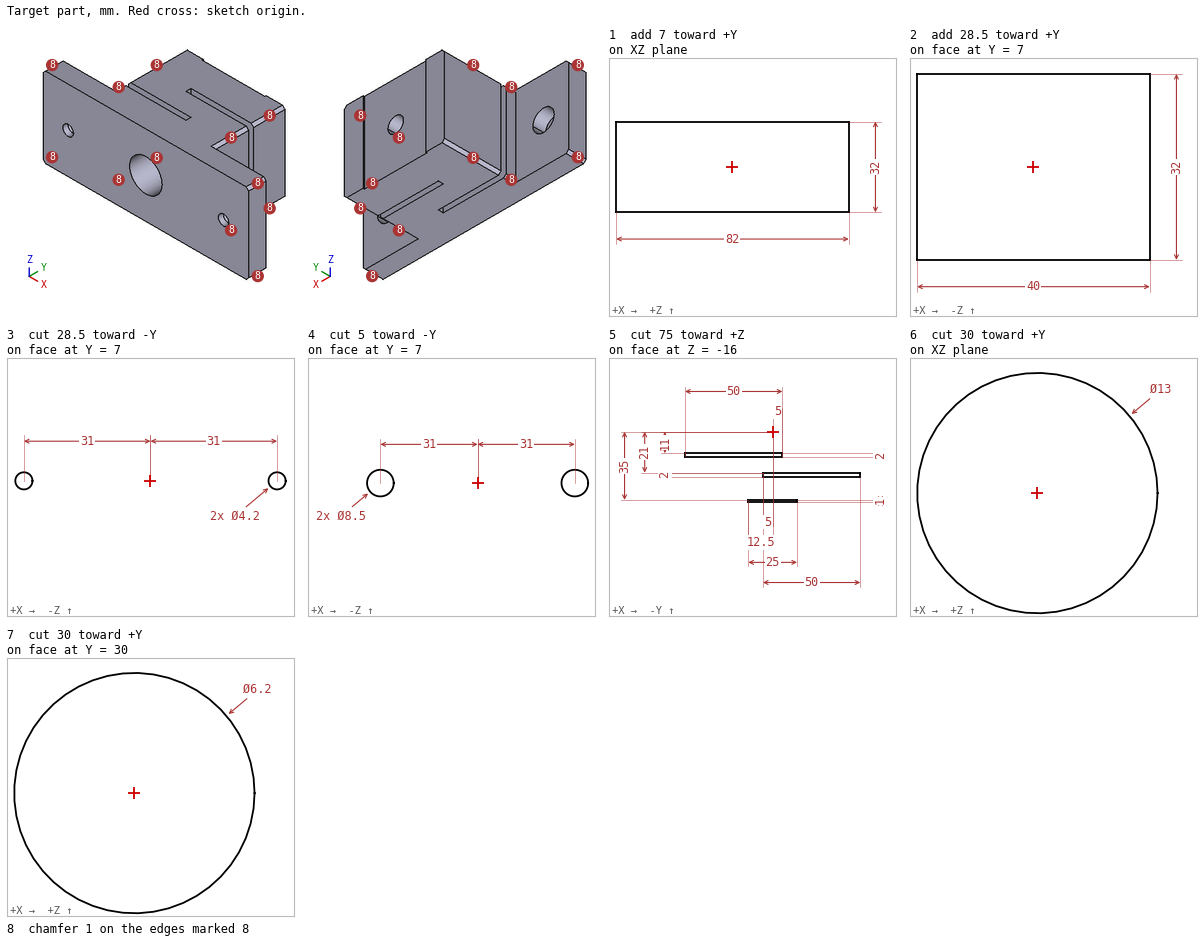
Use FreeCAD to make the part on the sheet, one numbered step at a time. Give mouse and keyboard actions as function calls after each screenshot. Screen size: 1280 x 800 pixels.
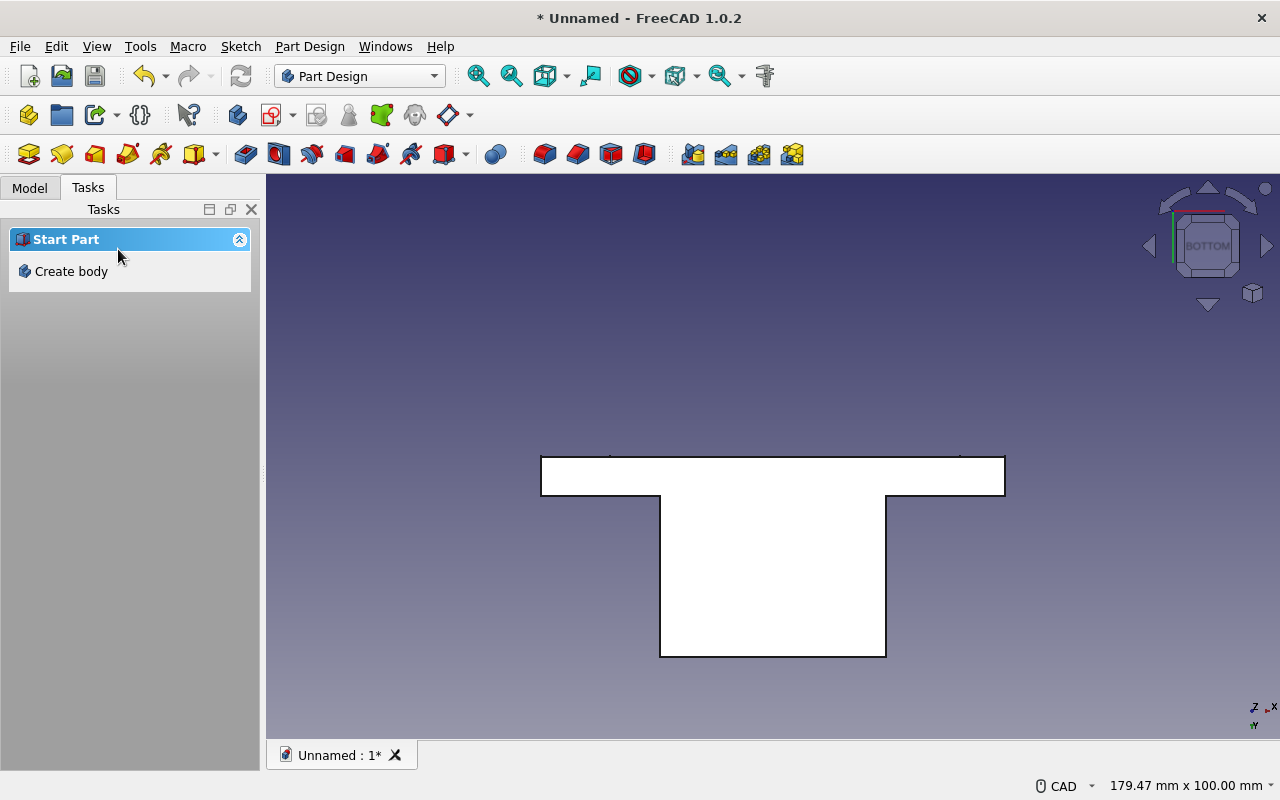
click(773, 556)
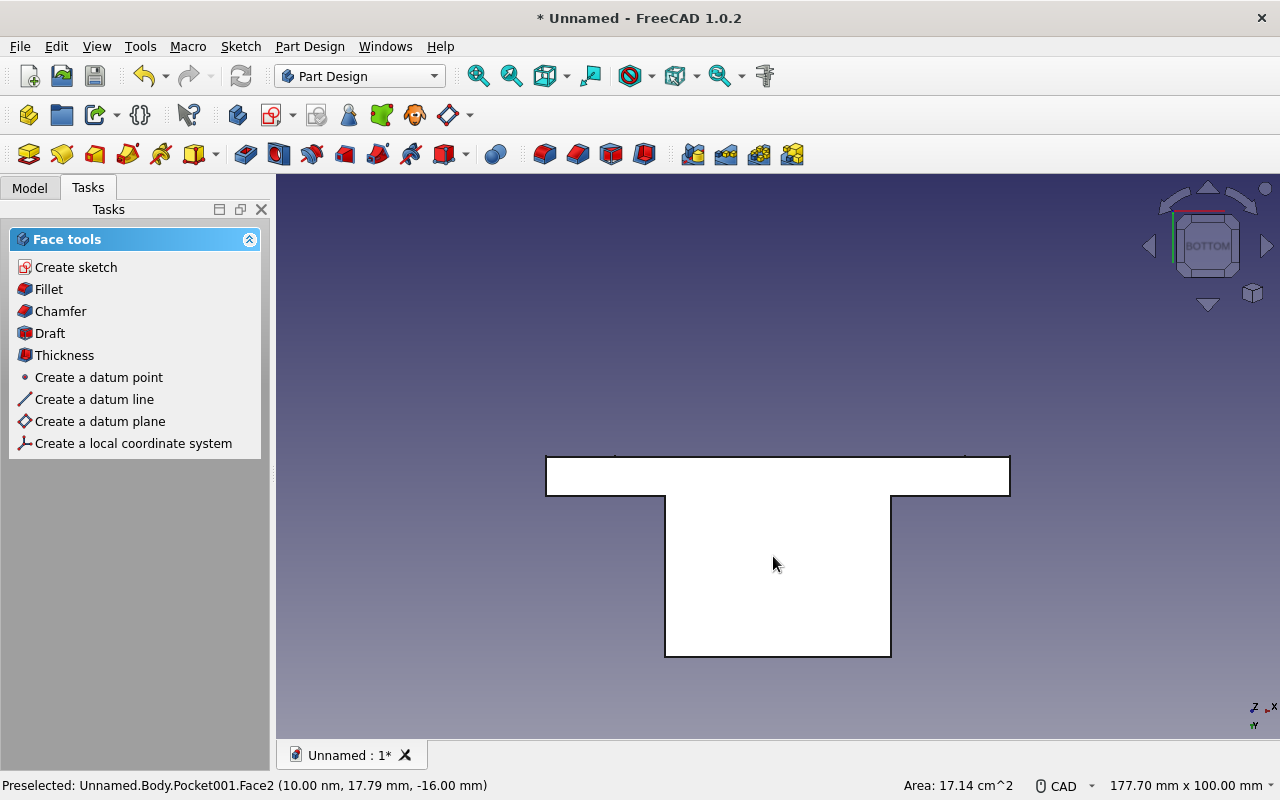
click(270, 116)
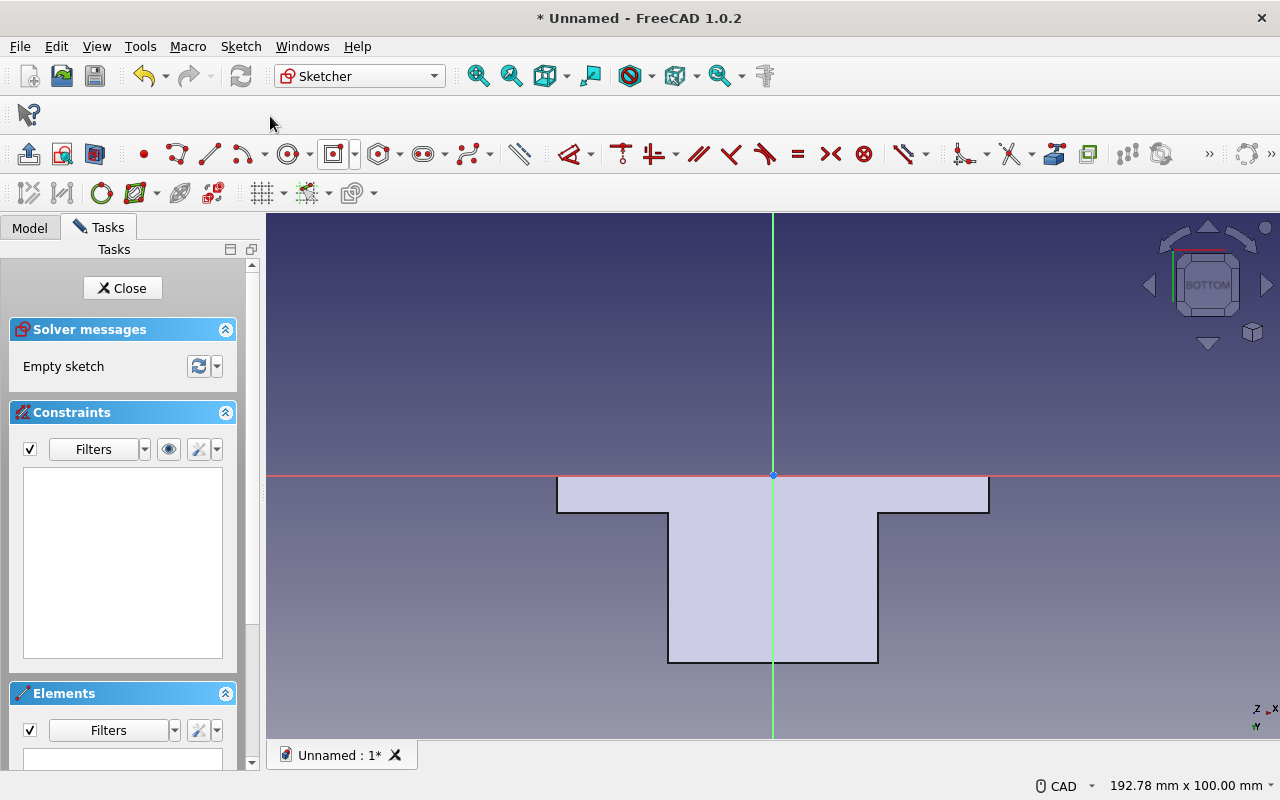
key(g)
key(r)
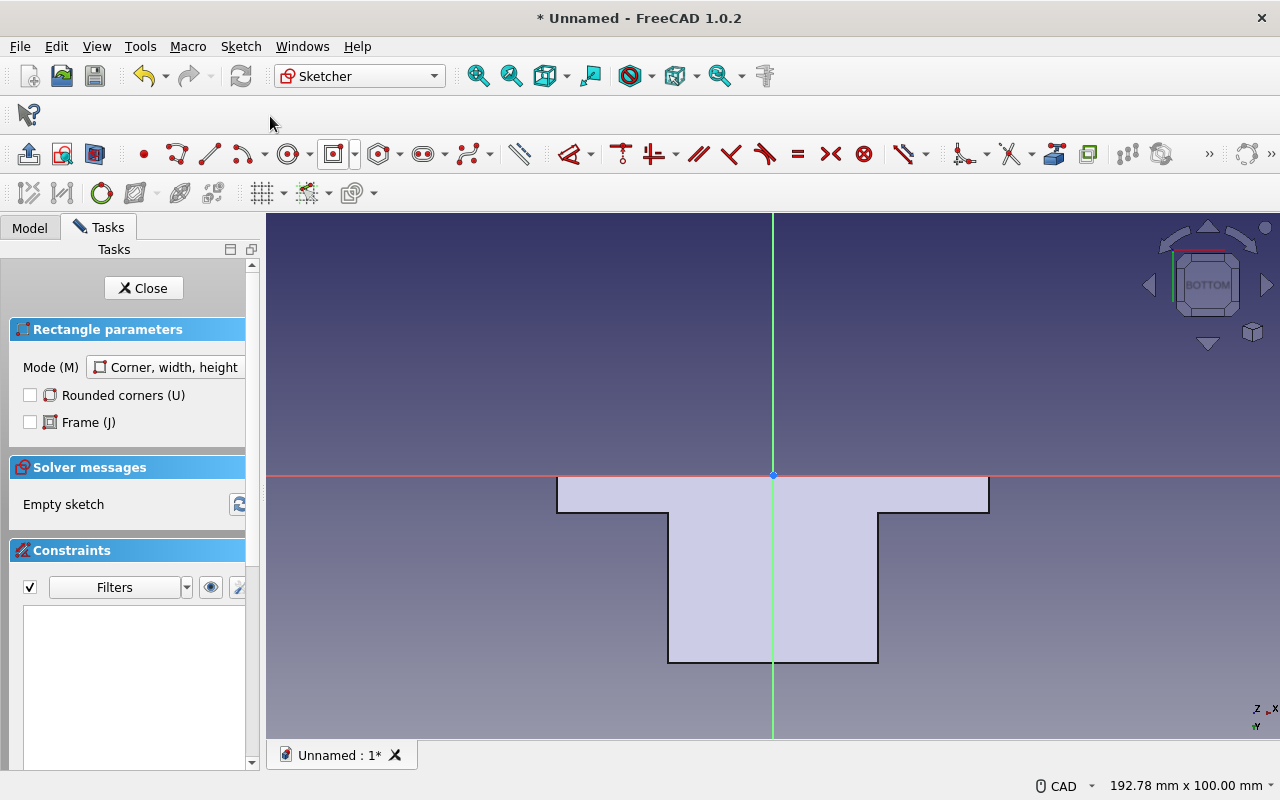
scroll(536, 534, up, 3)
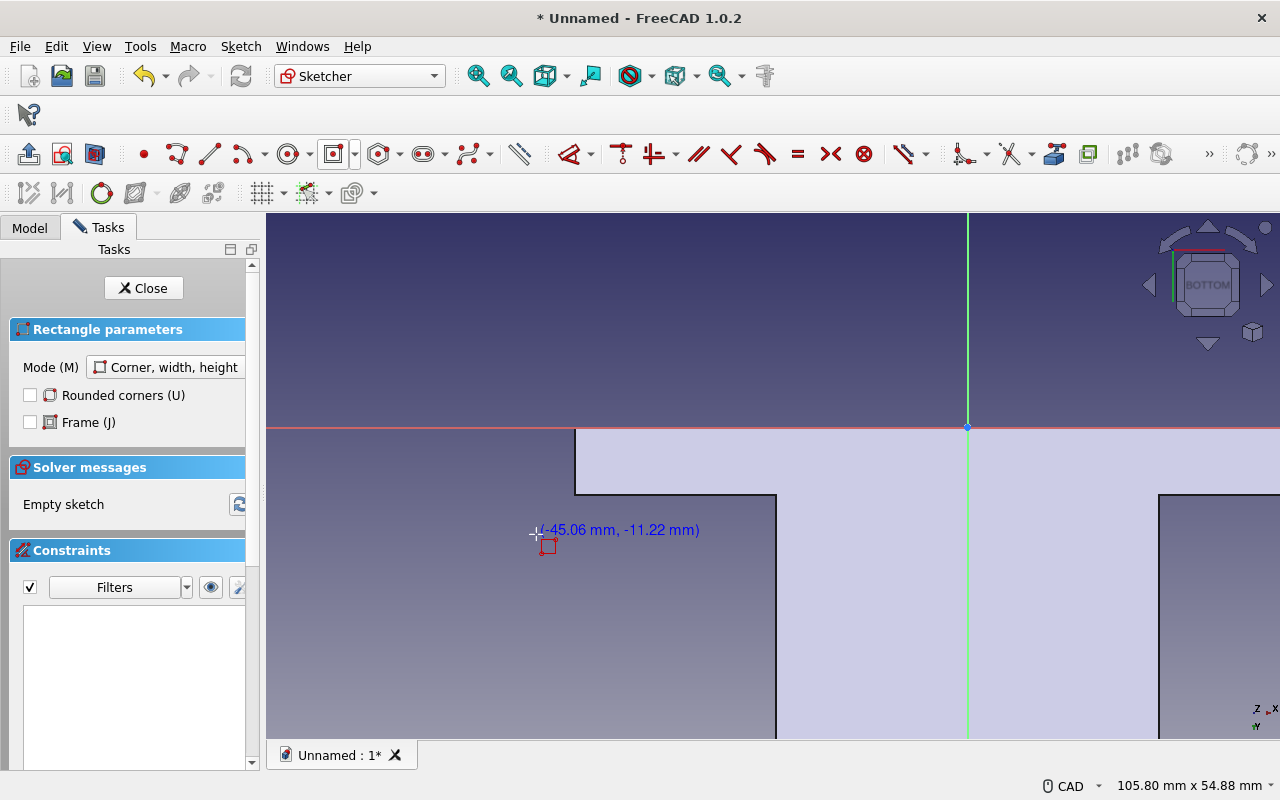
click(536, 533)
move(1016, 552)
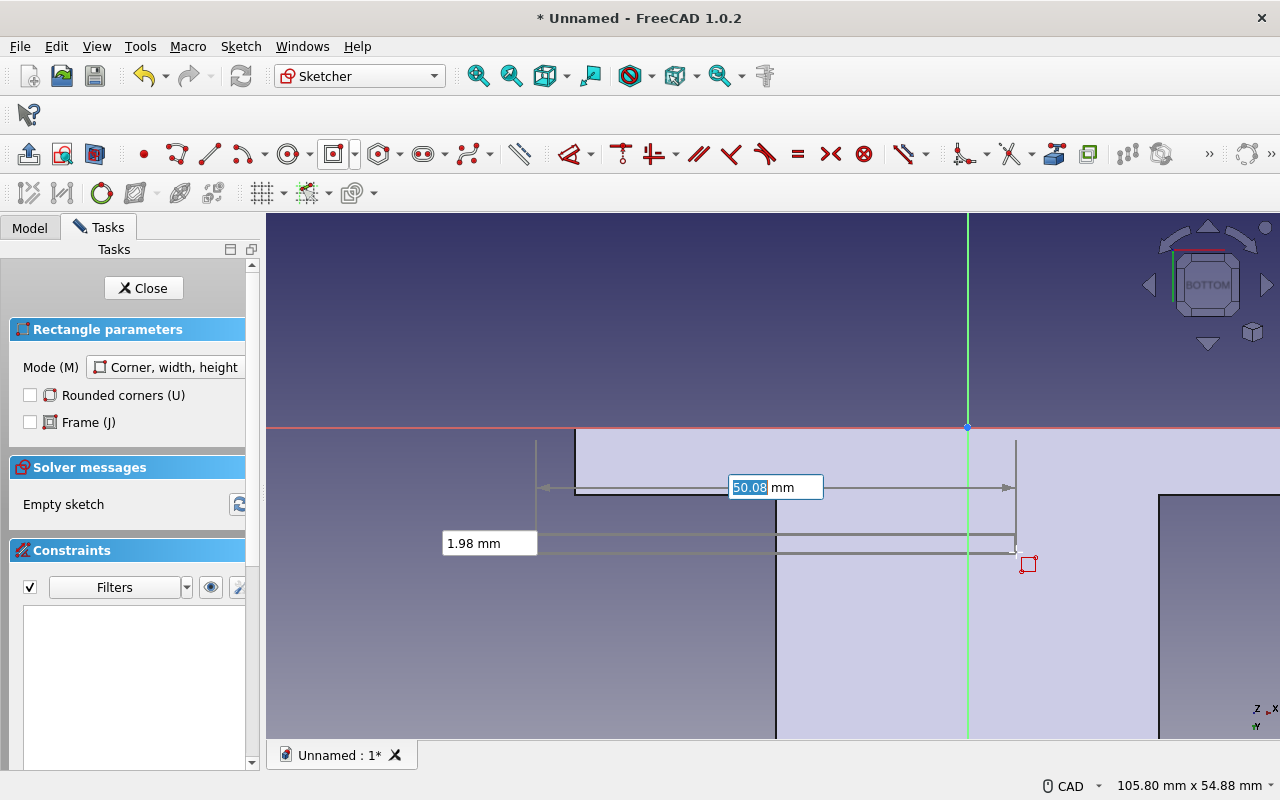
text(50)
key(Tab)
text(2)
key(Return)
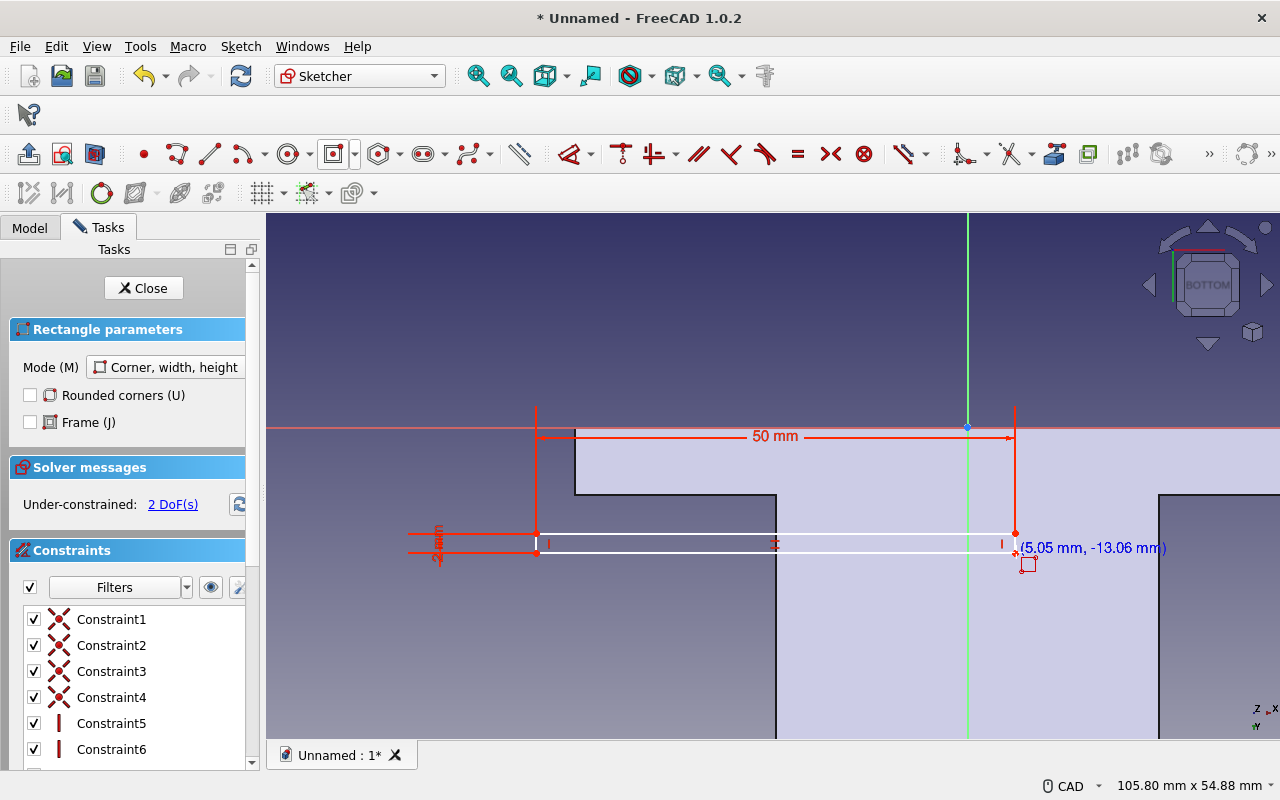
click(920, 629)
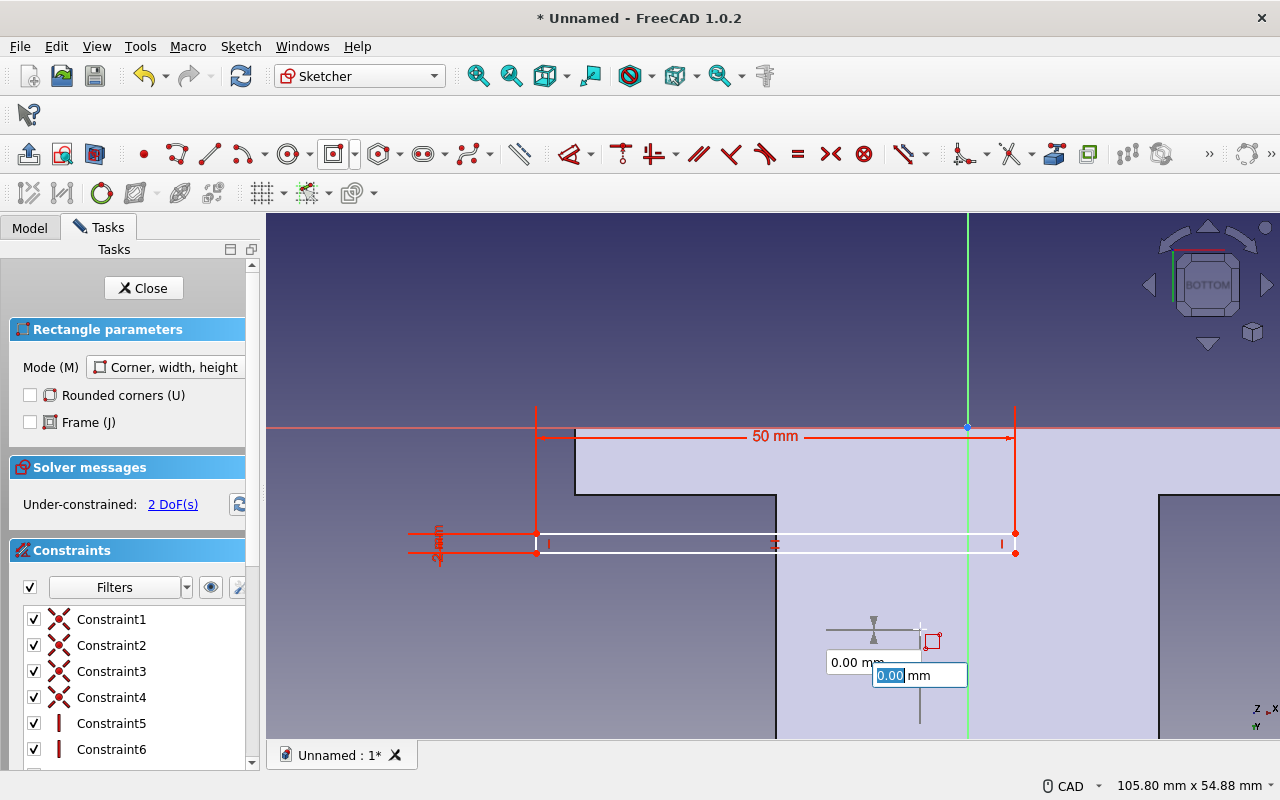
scroll(294, 241, down, 2)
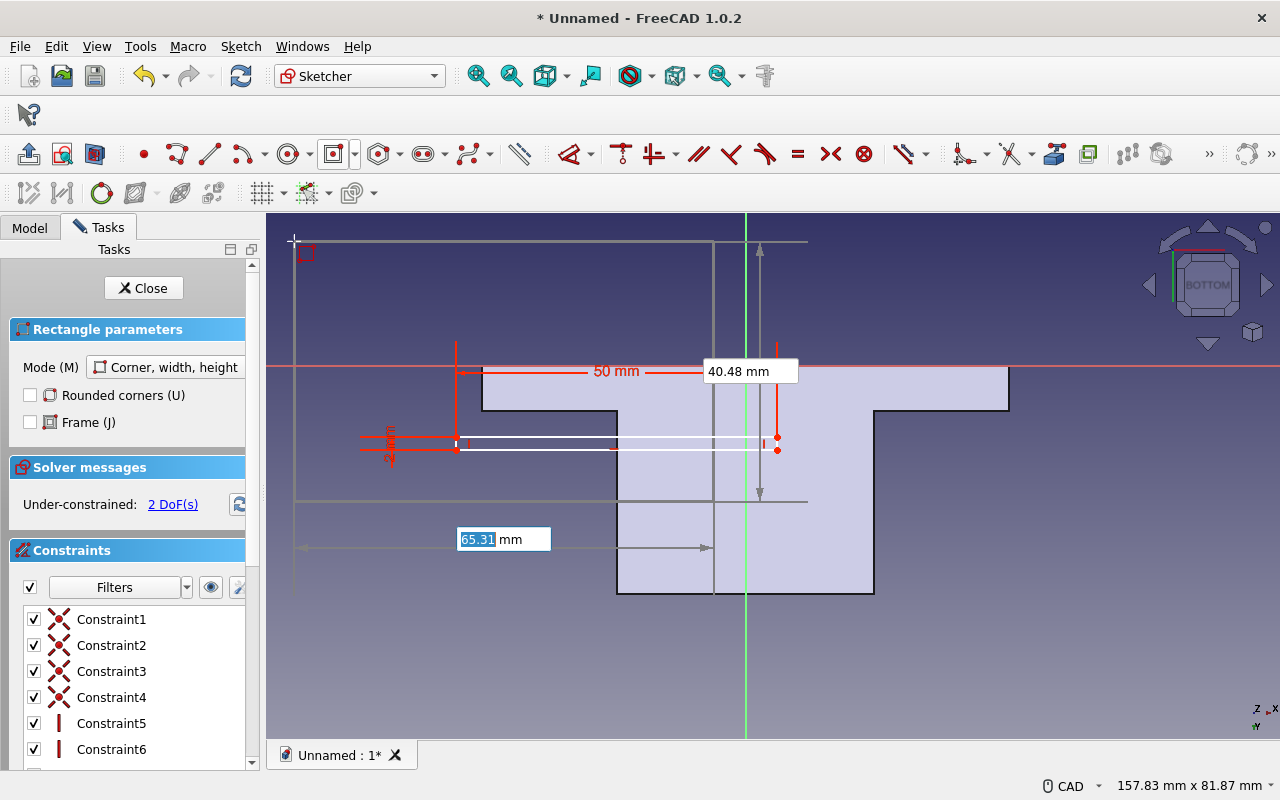
click(1035, 514)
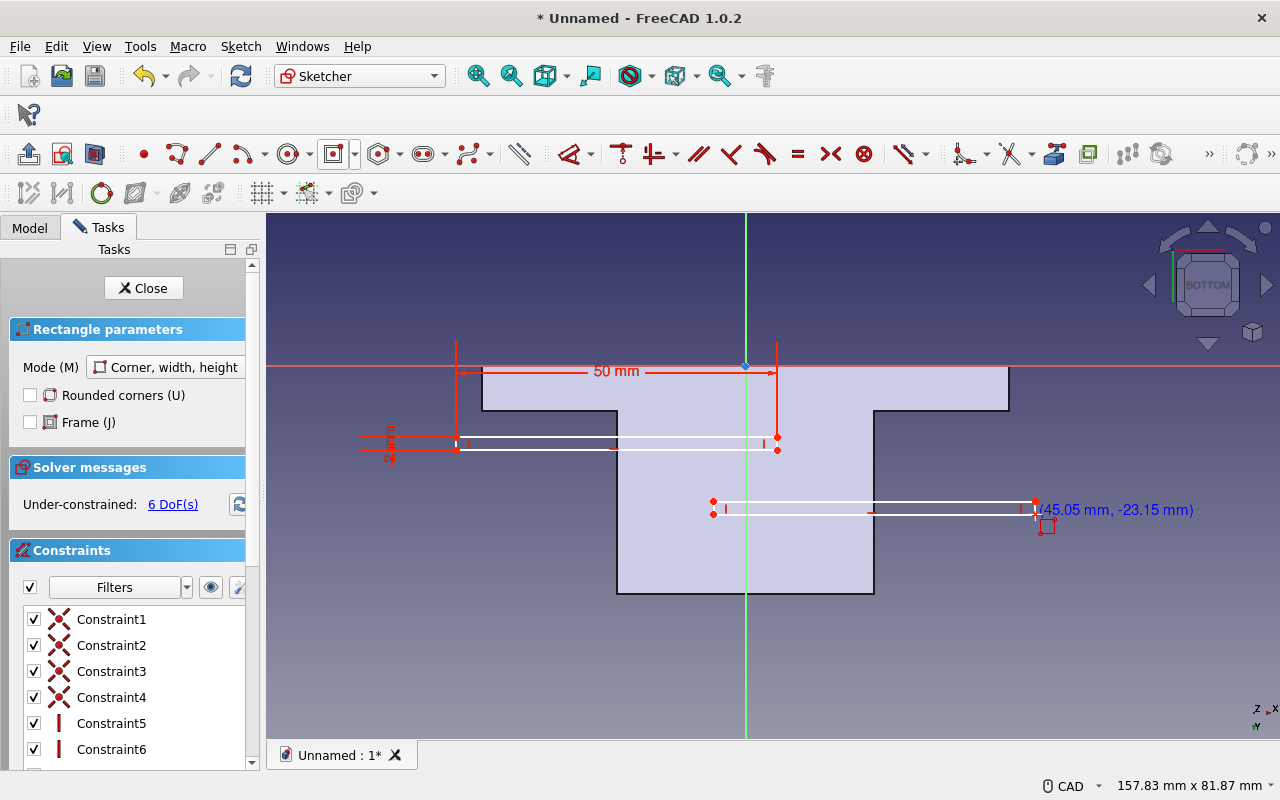
scroll(665, 591, up, 5)